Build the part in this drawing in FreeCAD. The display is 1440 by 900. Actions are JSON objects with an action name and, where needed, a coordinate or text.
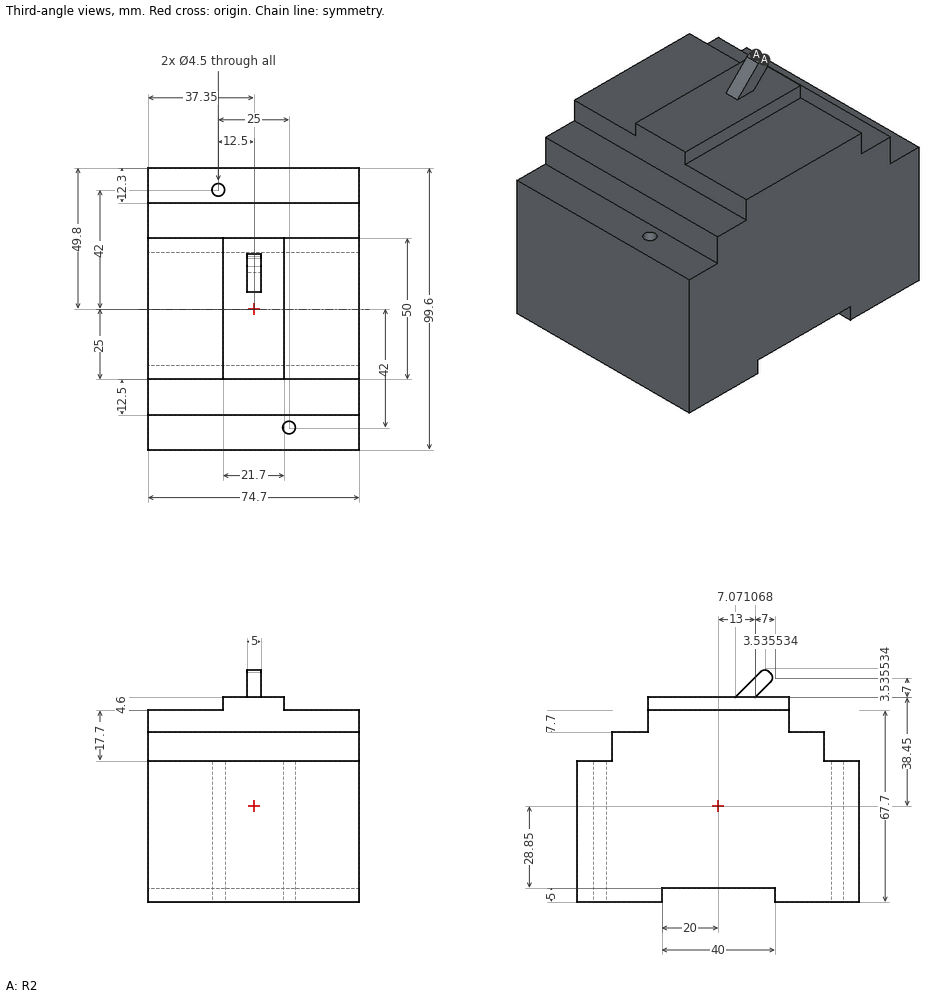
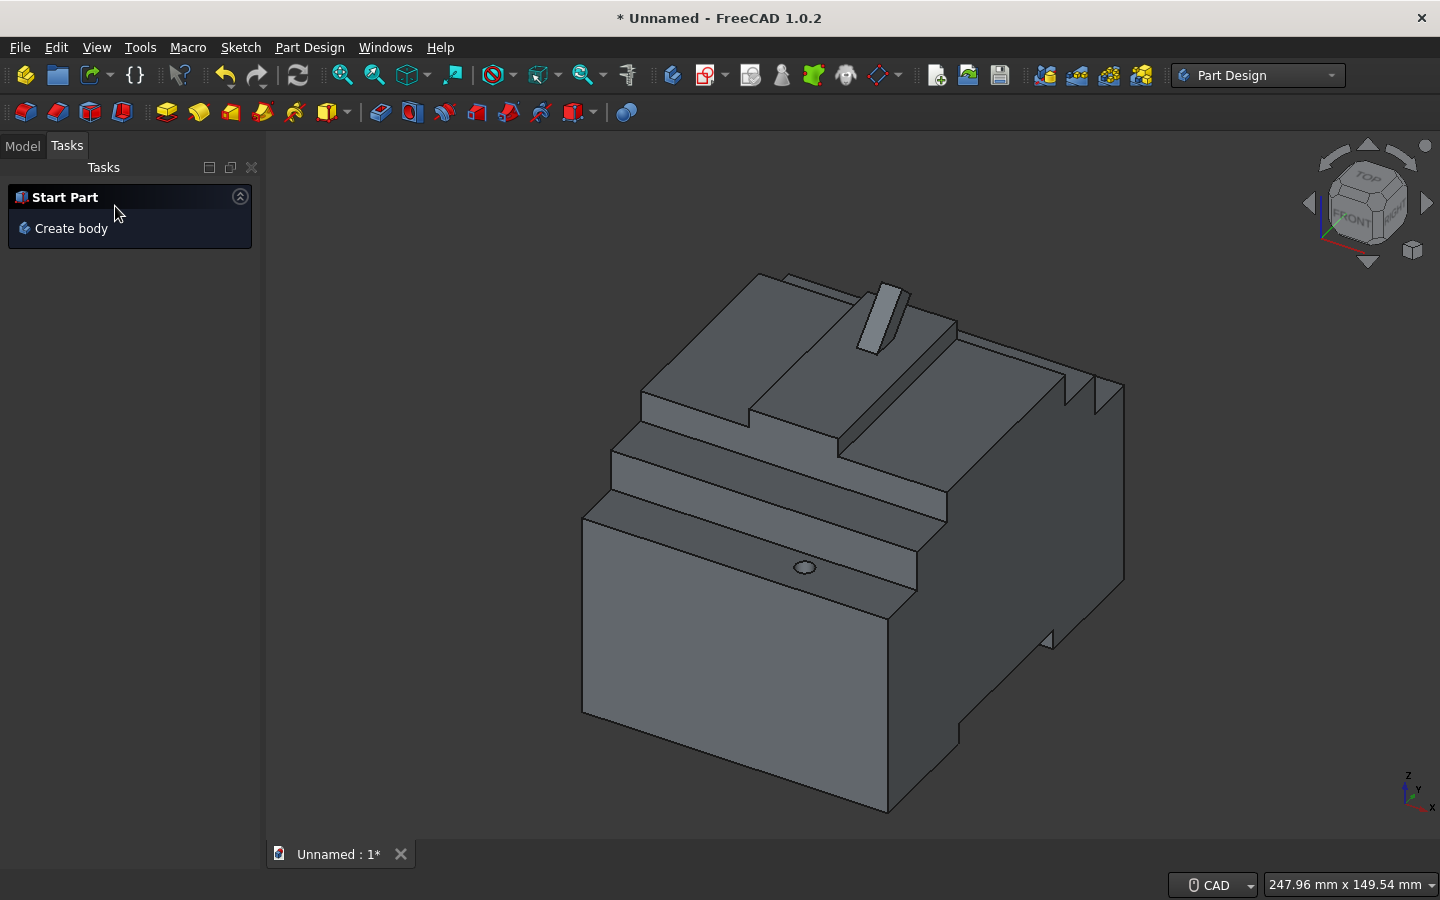
{"action": "key", "text": "0"}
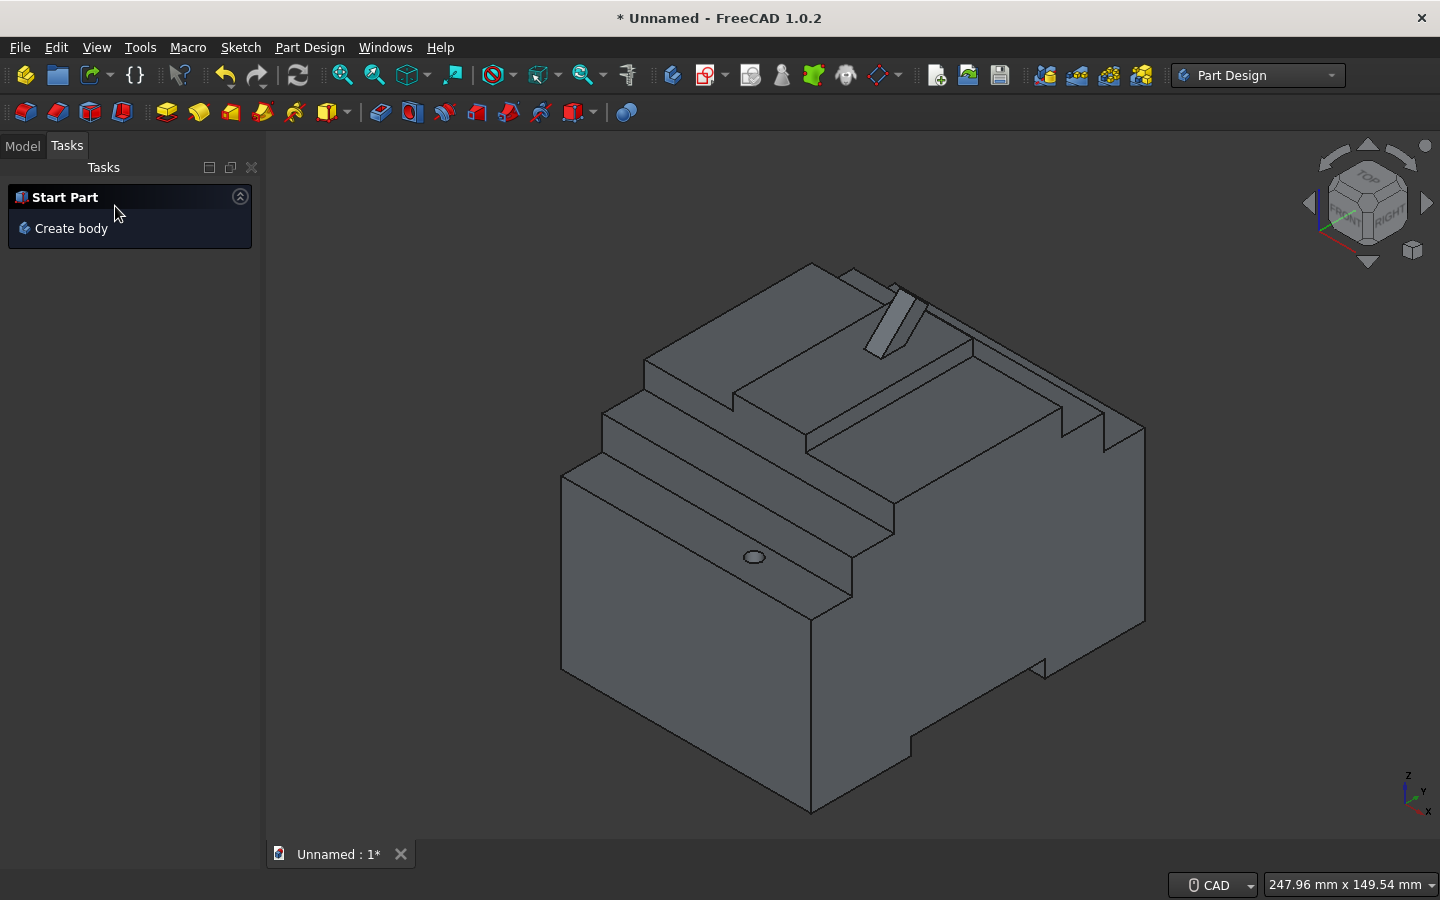
{"action": "left_click", "coordinate": [908, 292]}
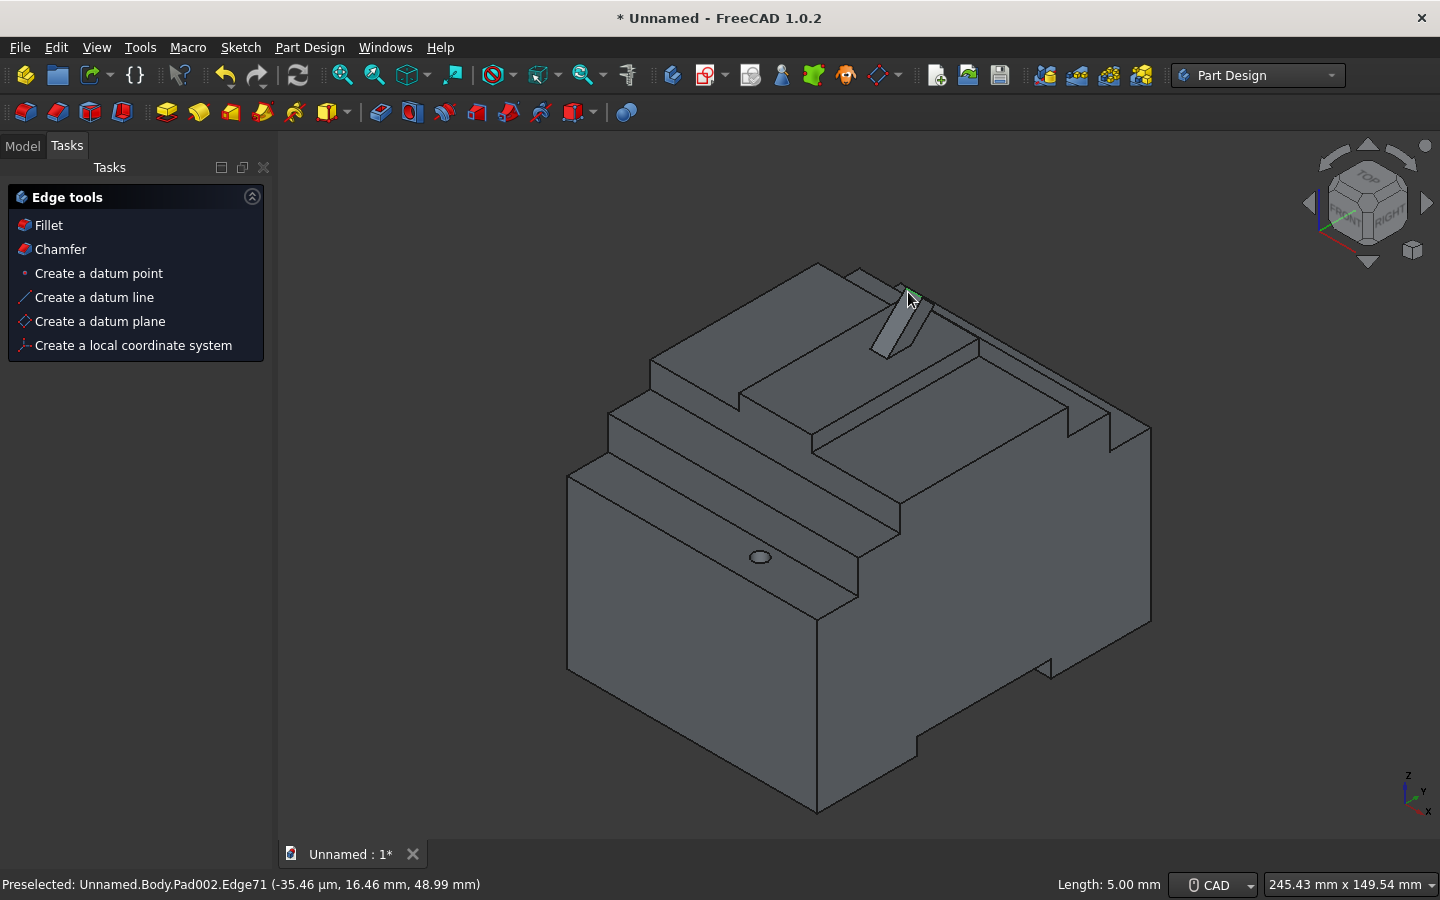
{"action": "key", "text": "2"}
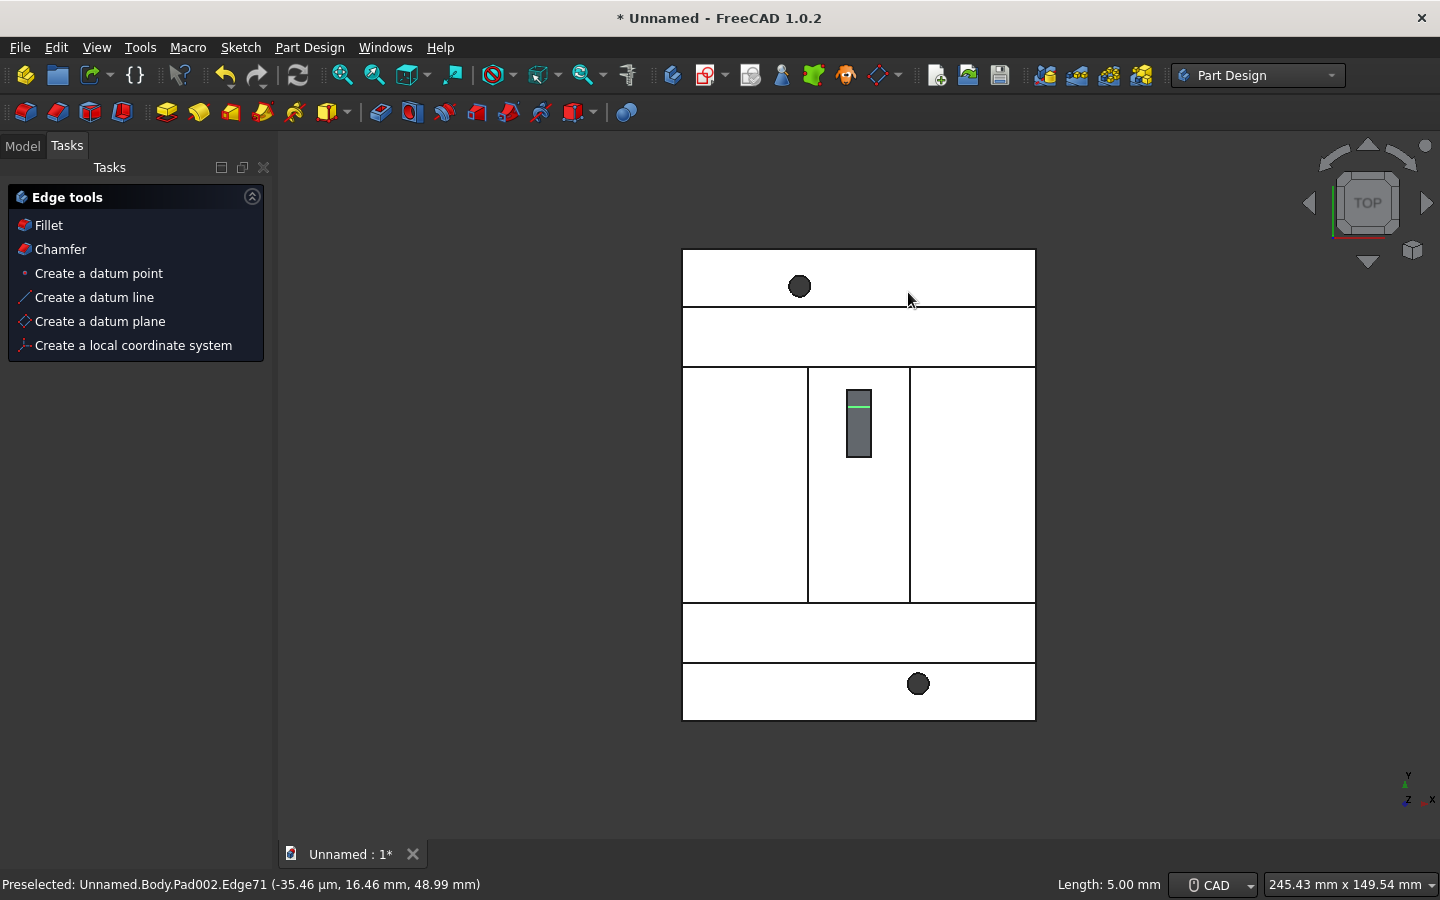
{"action": "key", "text": "1"}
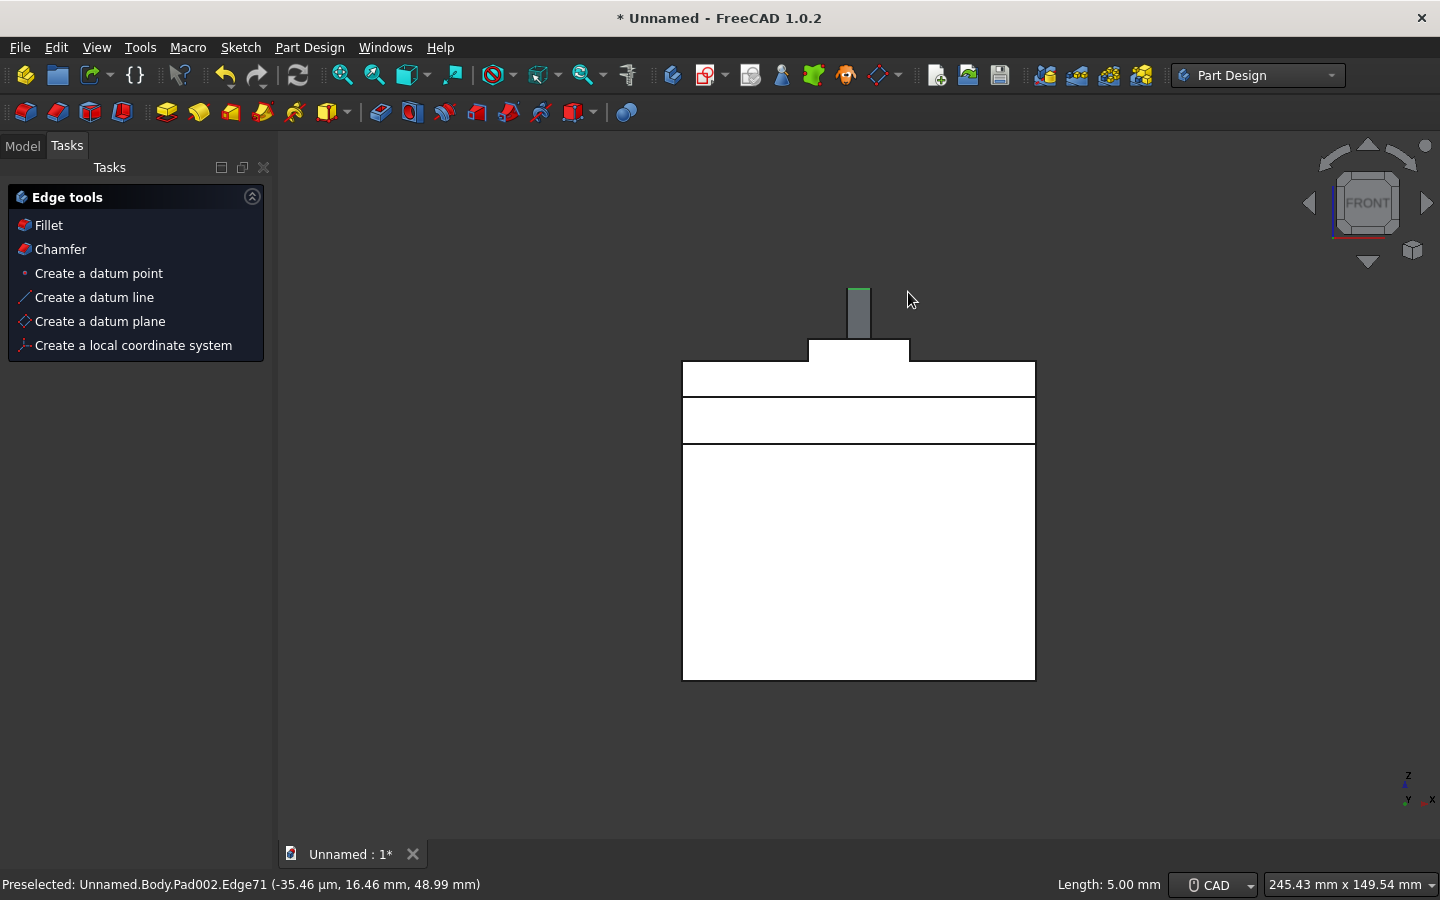
{"action": "key", "text": "3"}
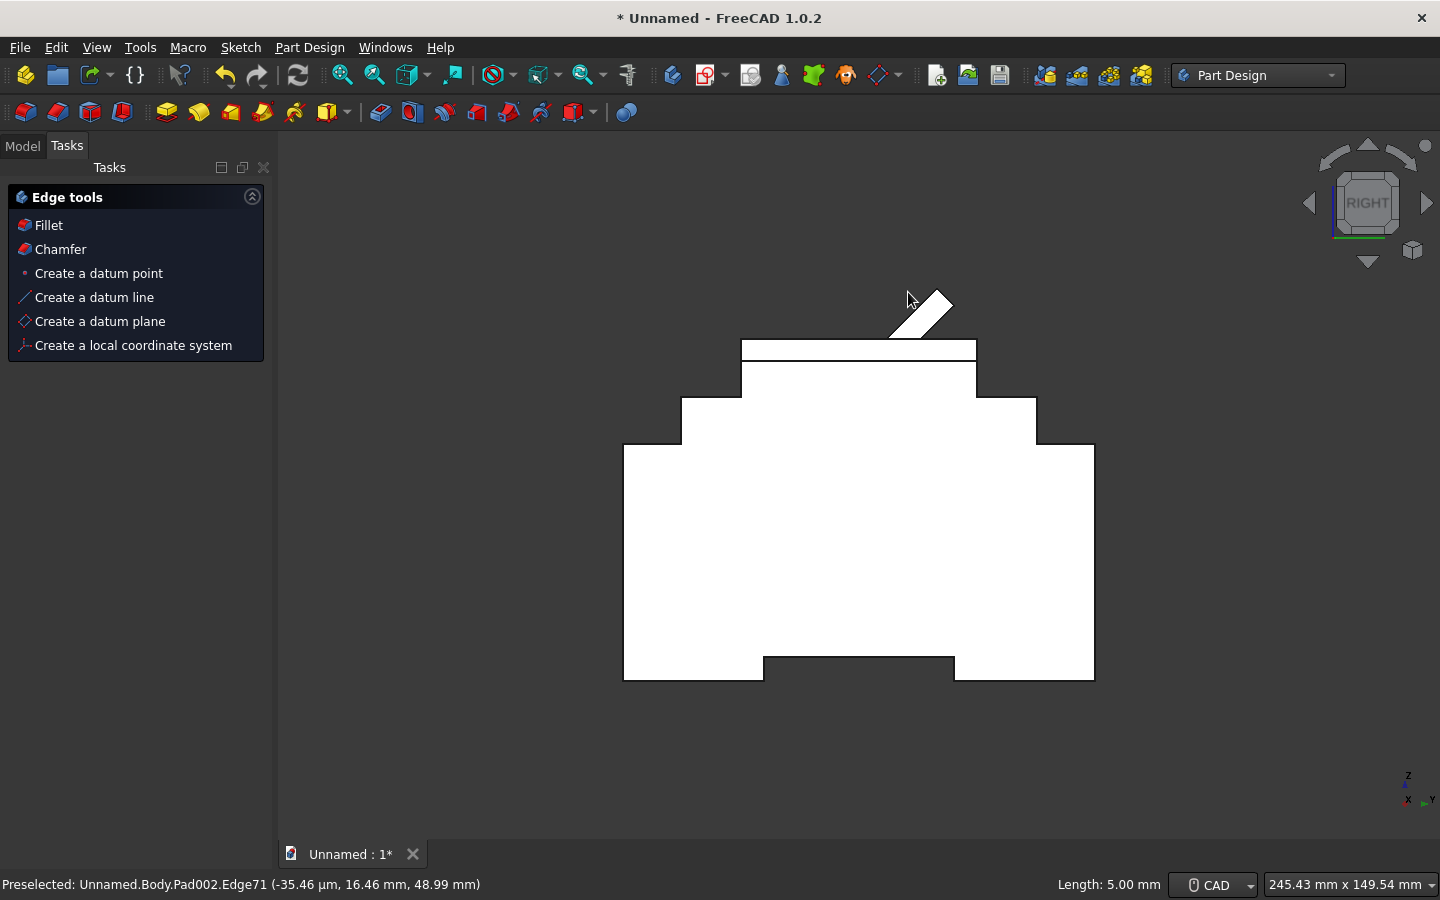
{"action": "key", "text": "5"}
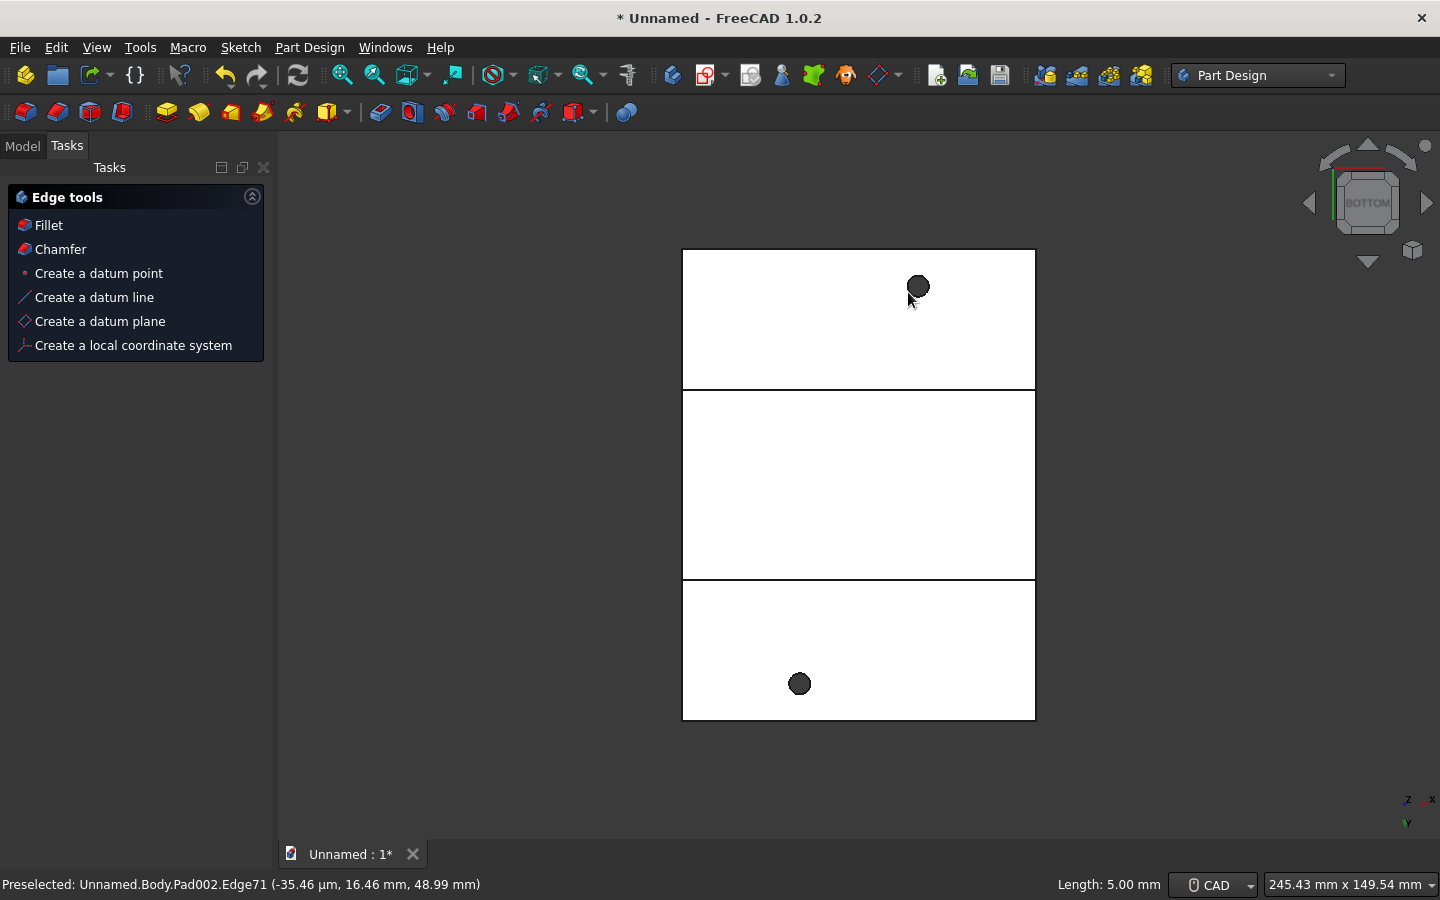
{"action": "key", "text": "4"}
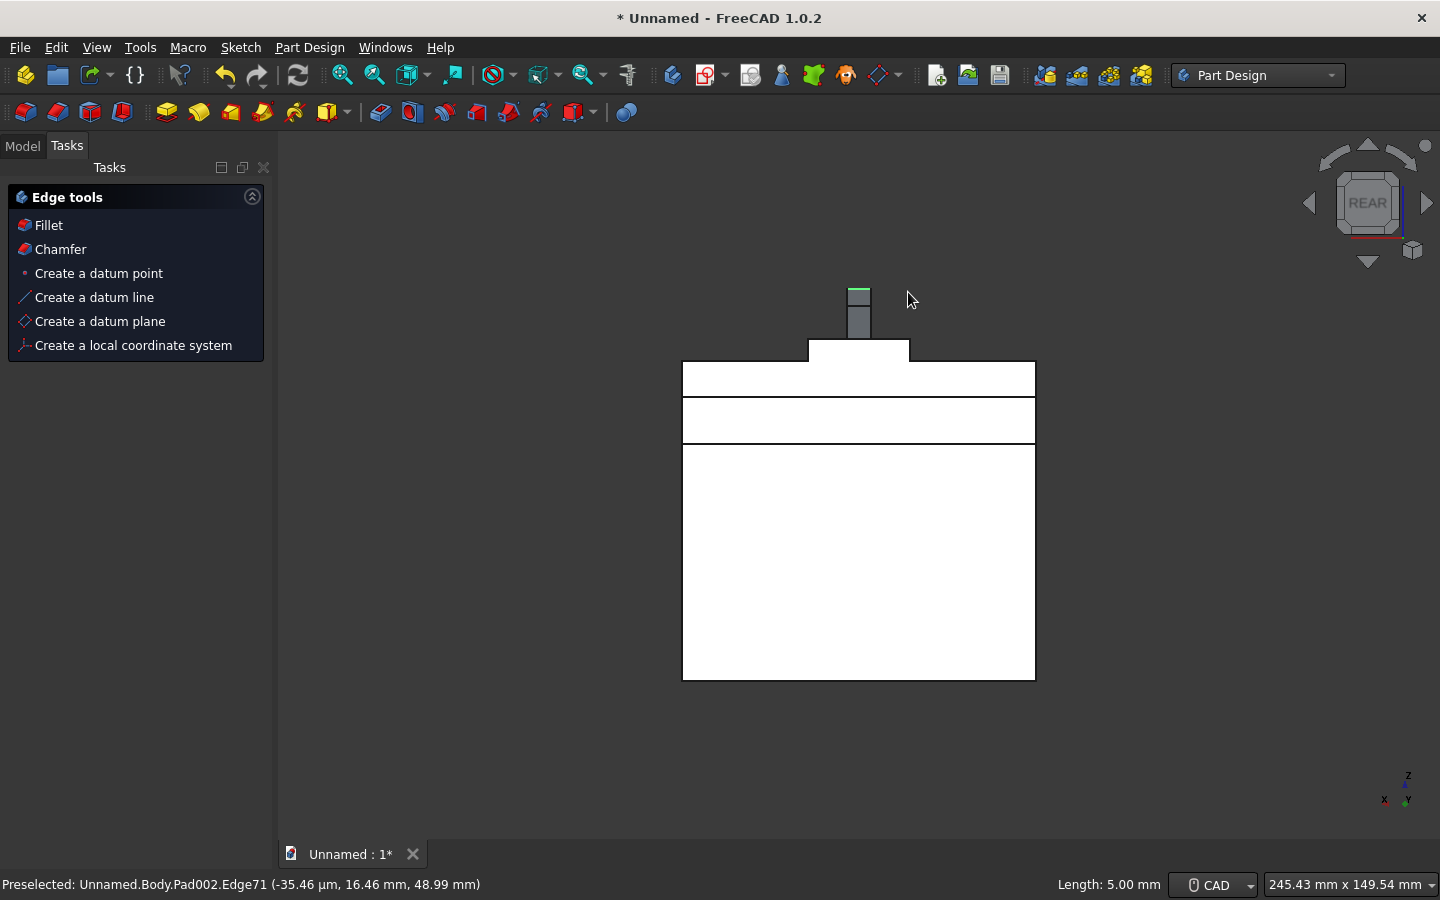
{"action": "left_click", "coordinate": [859, 305], "text": "ctrl"}